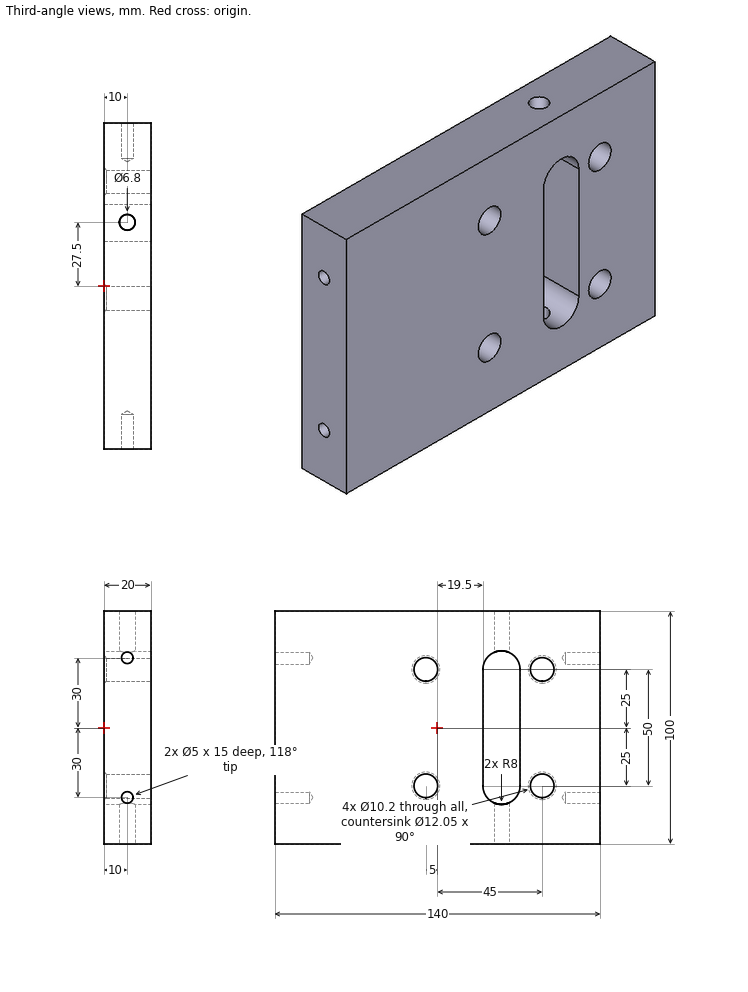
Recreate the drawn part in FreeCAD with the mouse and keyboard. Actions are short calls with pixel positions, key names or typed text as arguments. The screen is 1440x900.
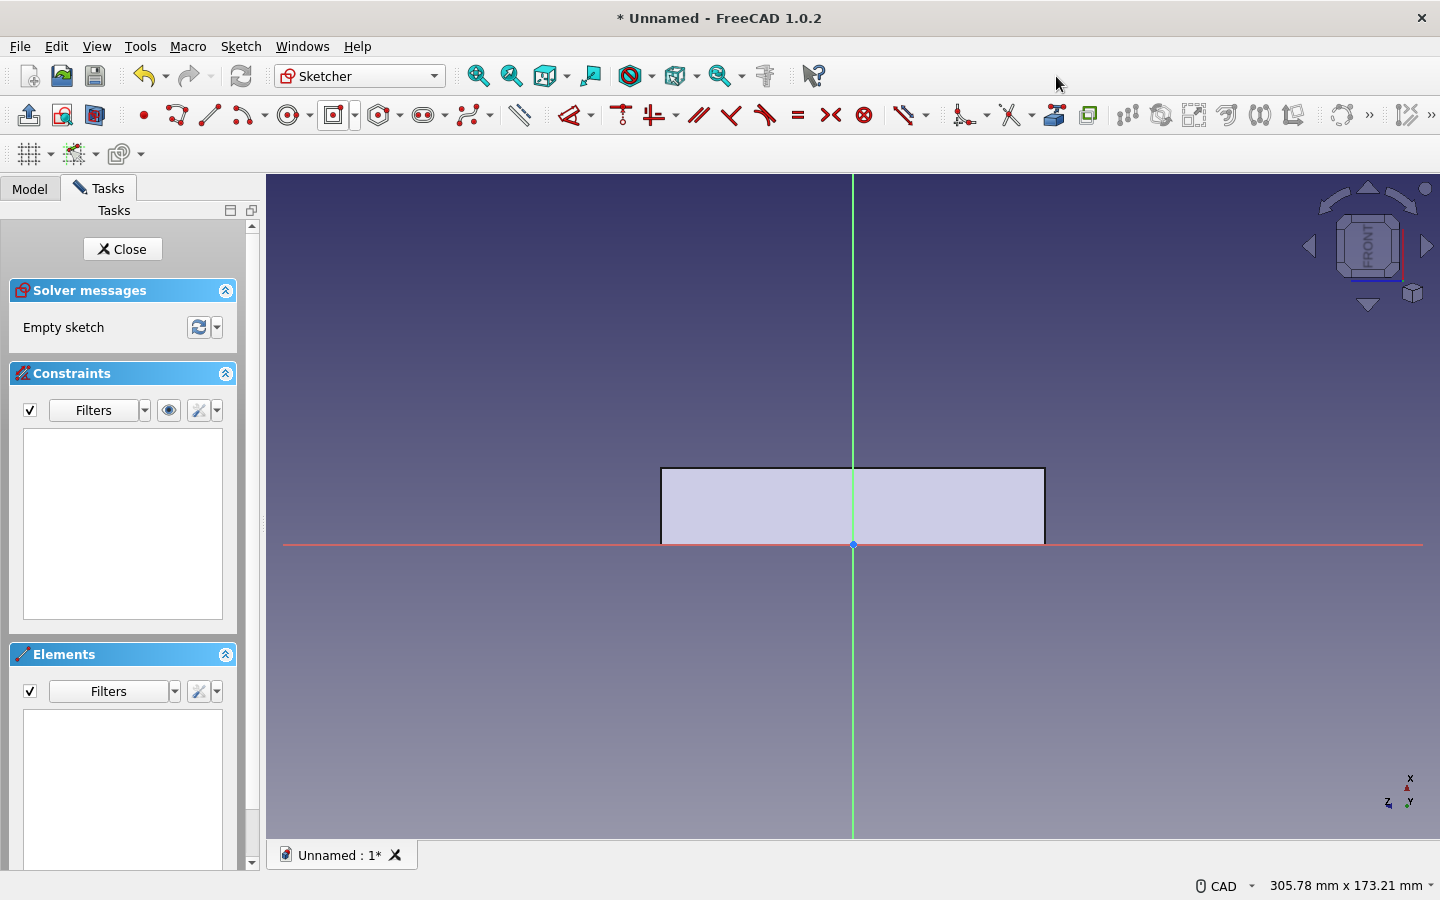
scroll(893, 529, up, 5)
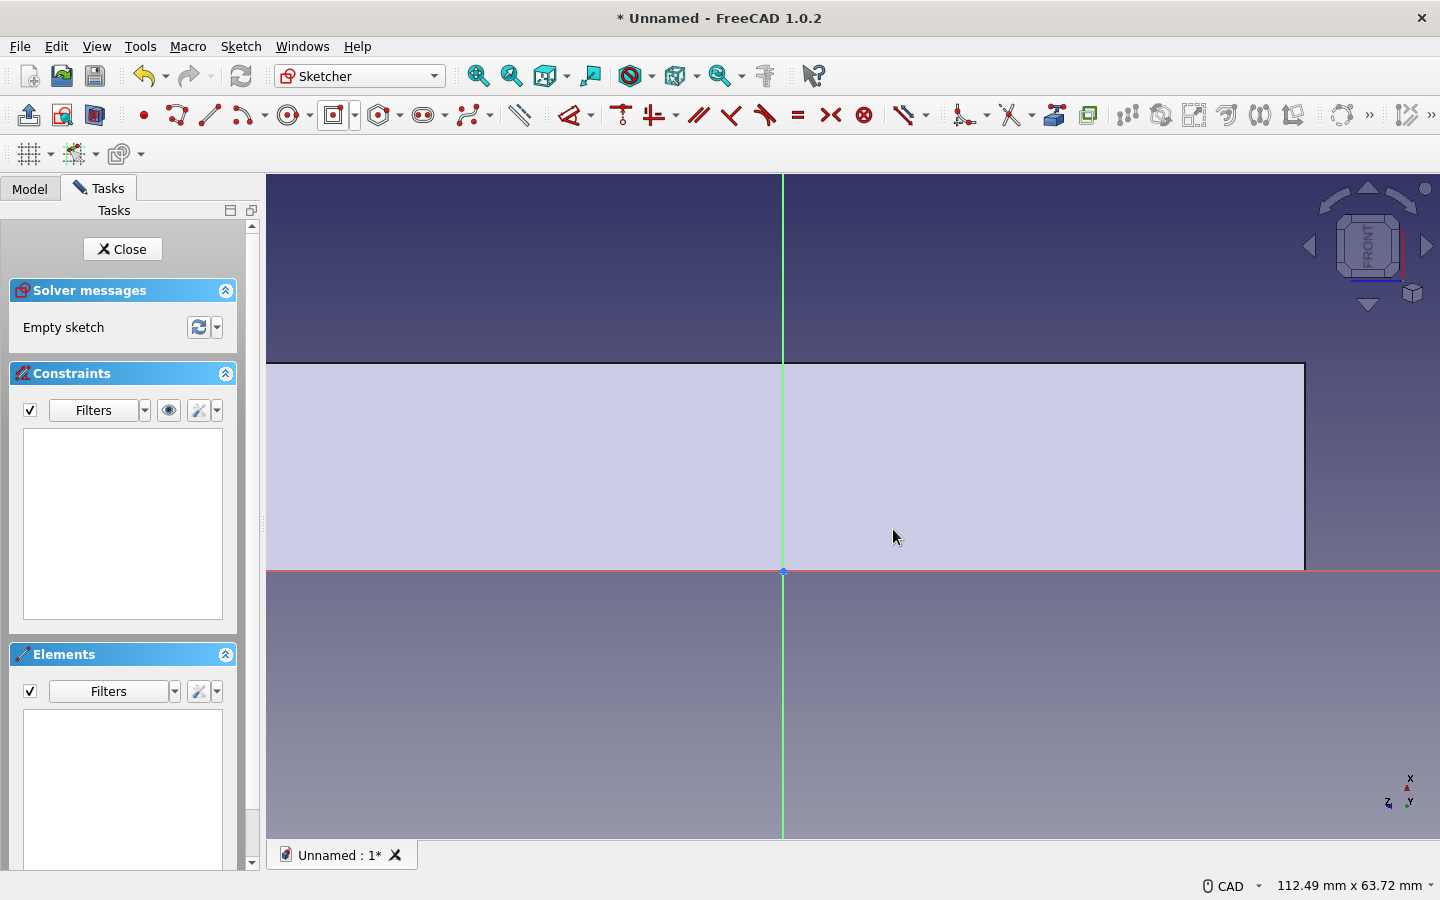
click(288, 116)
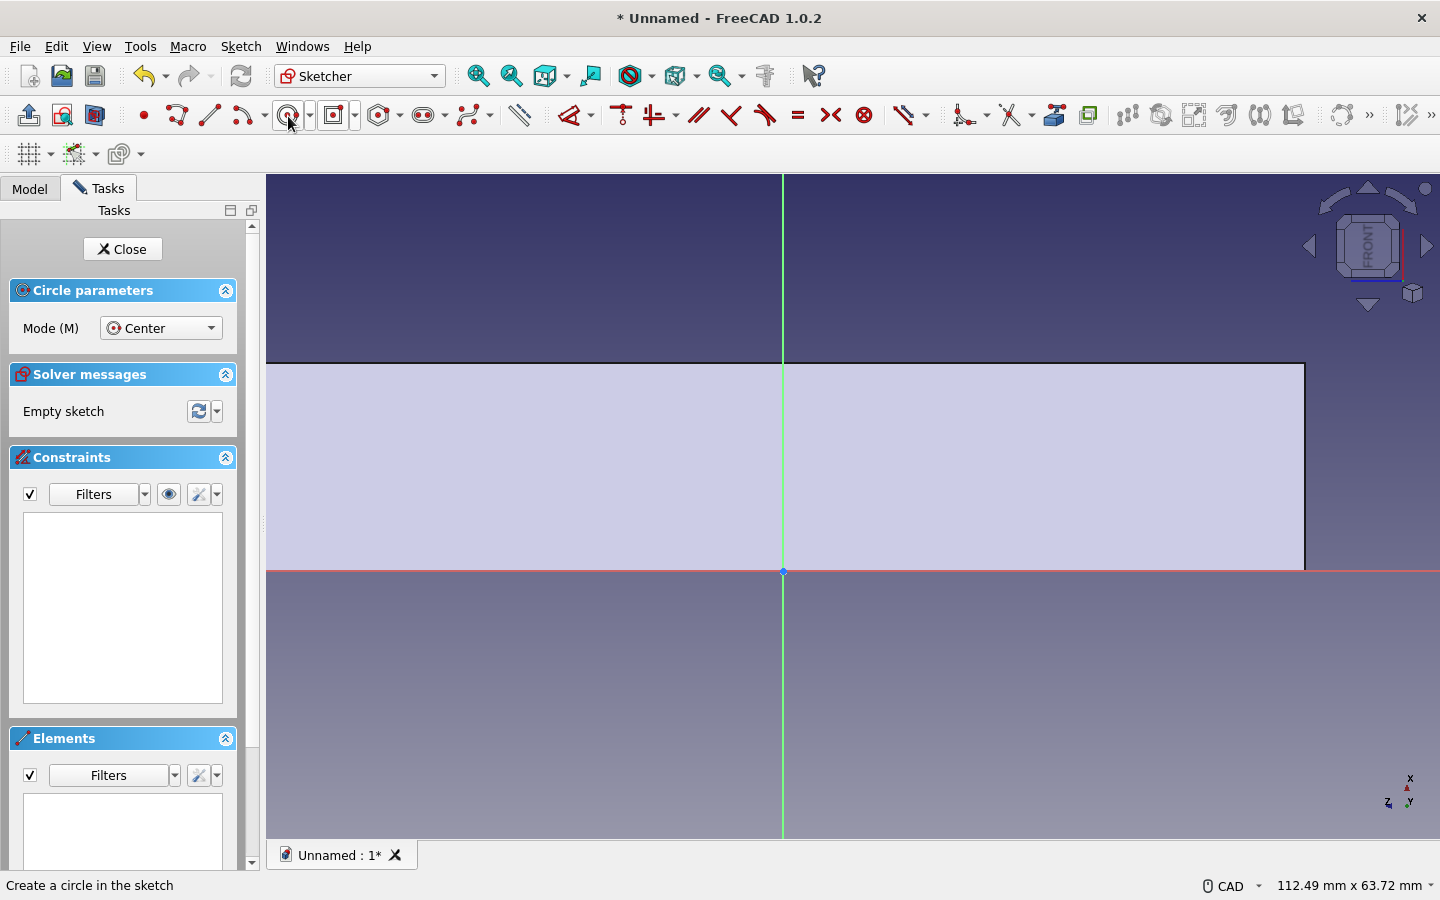
click(1096, 467)
move(1115, 448)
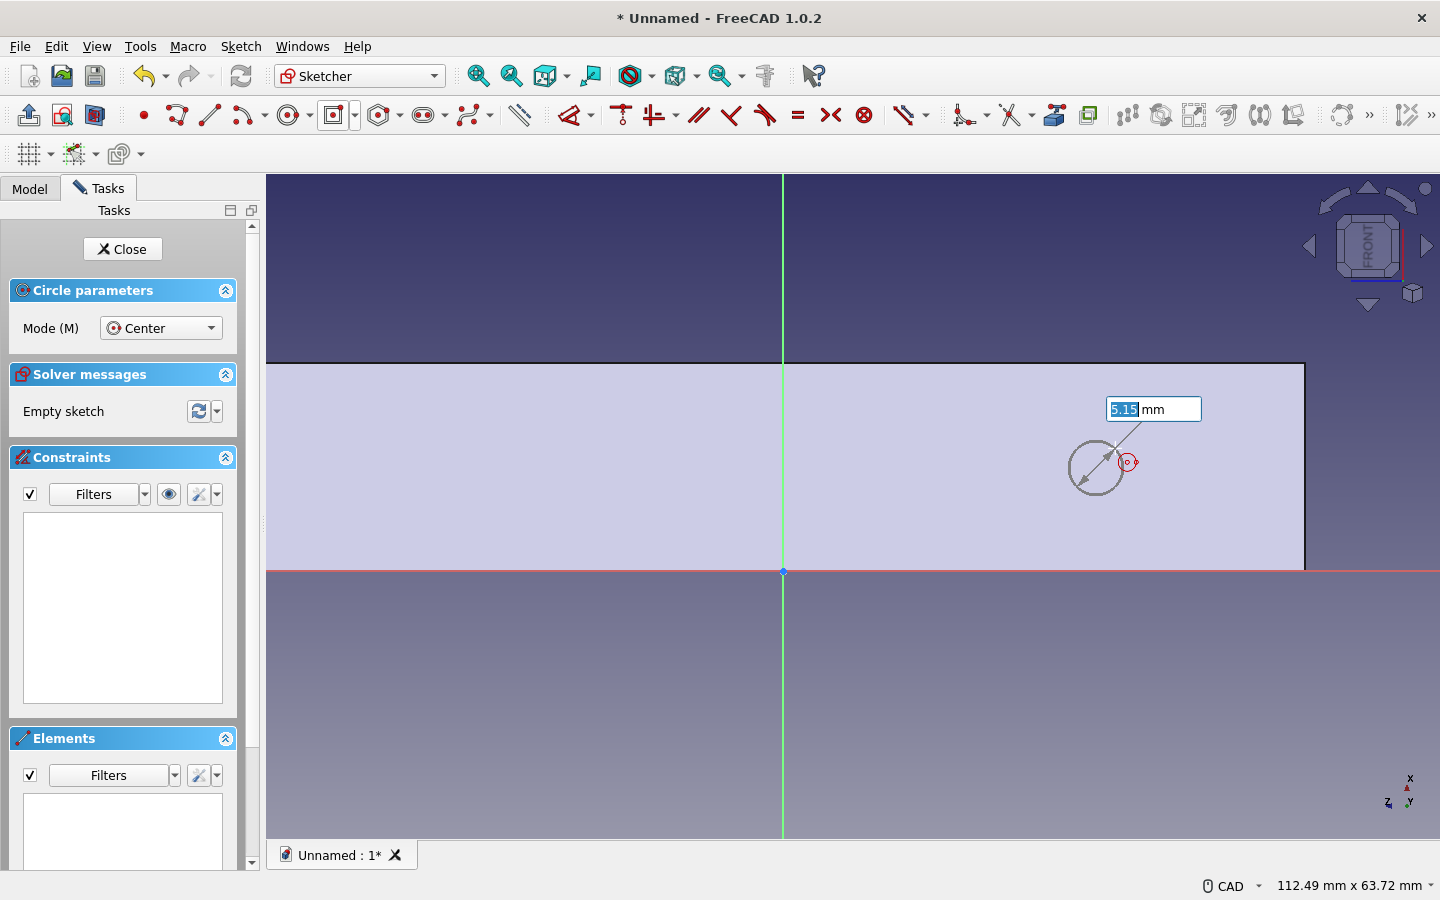
text(5)
key(Return)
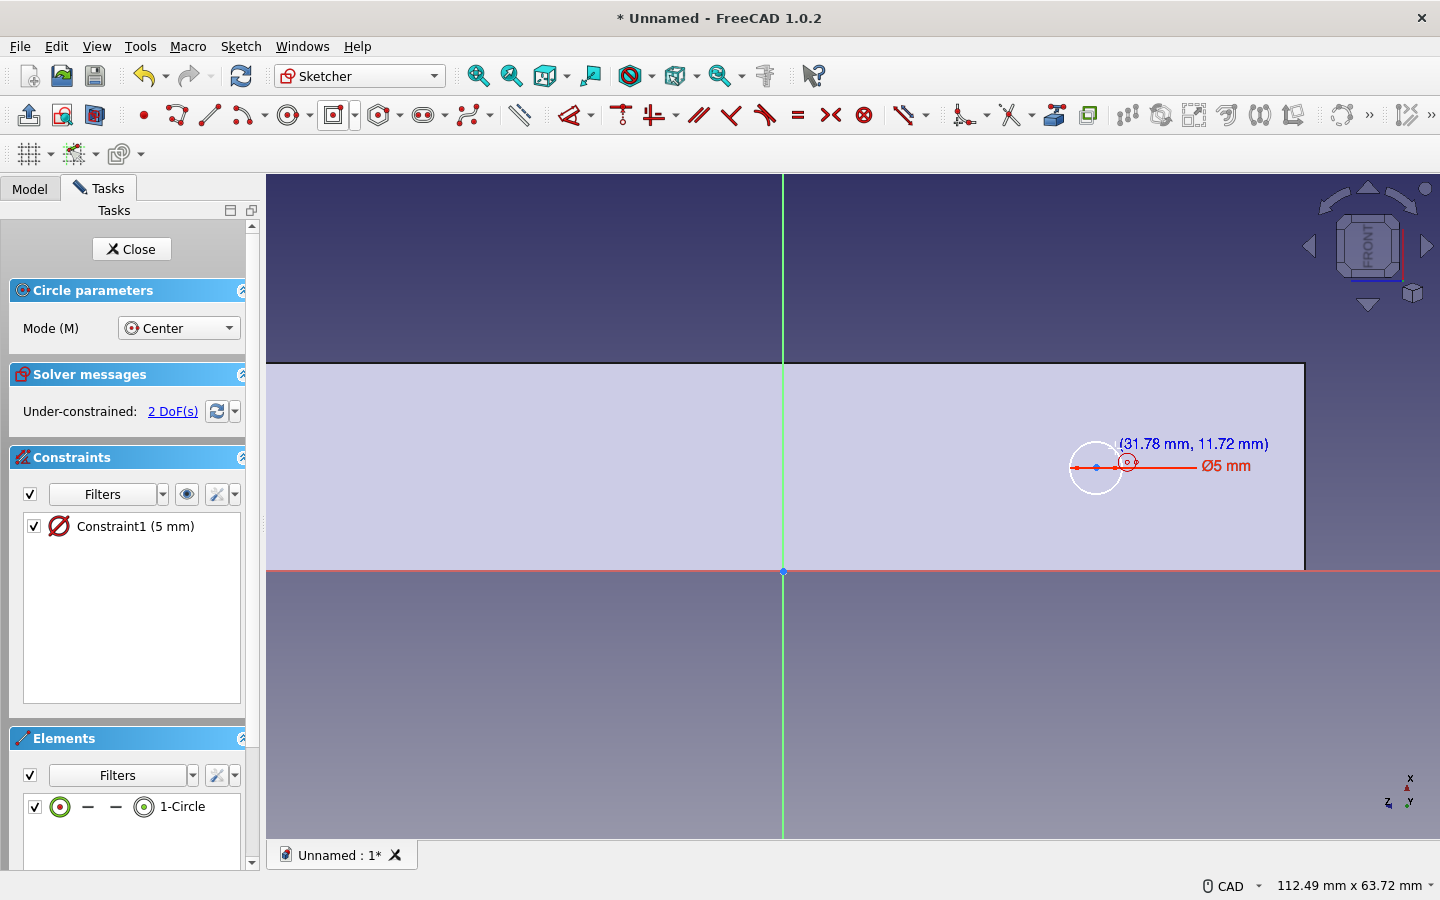
click(470, 467)
move(489, 448)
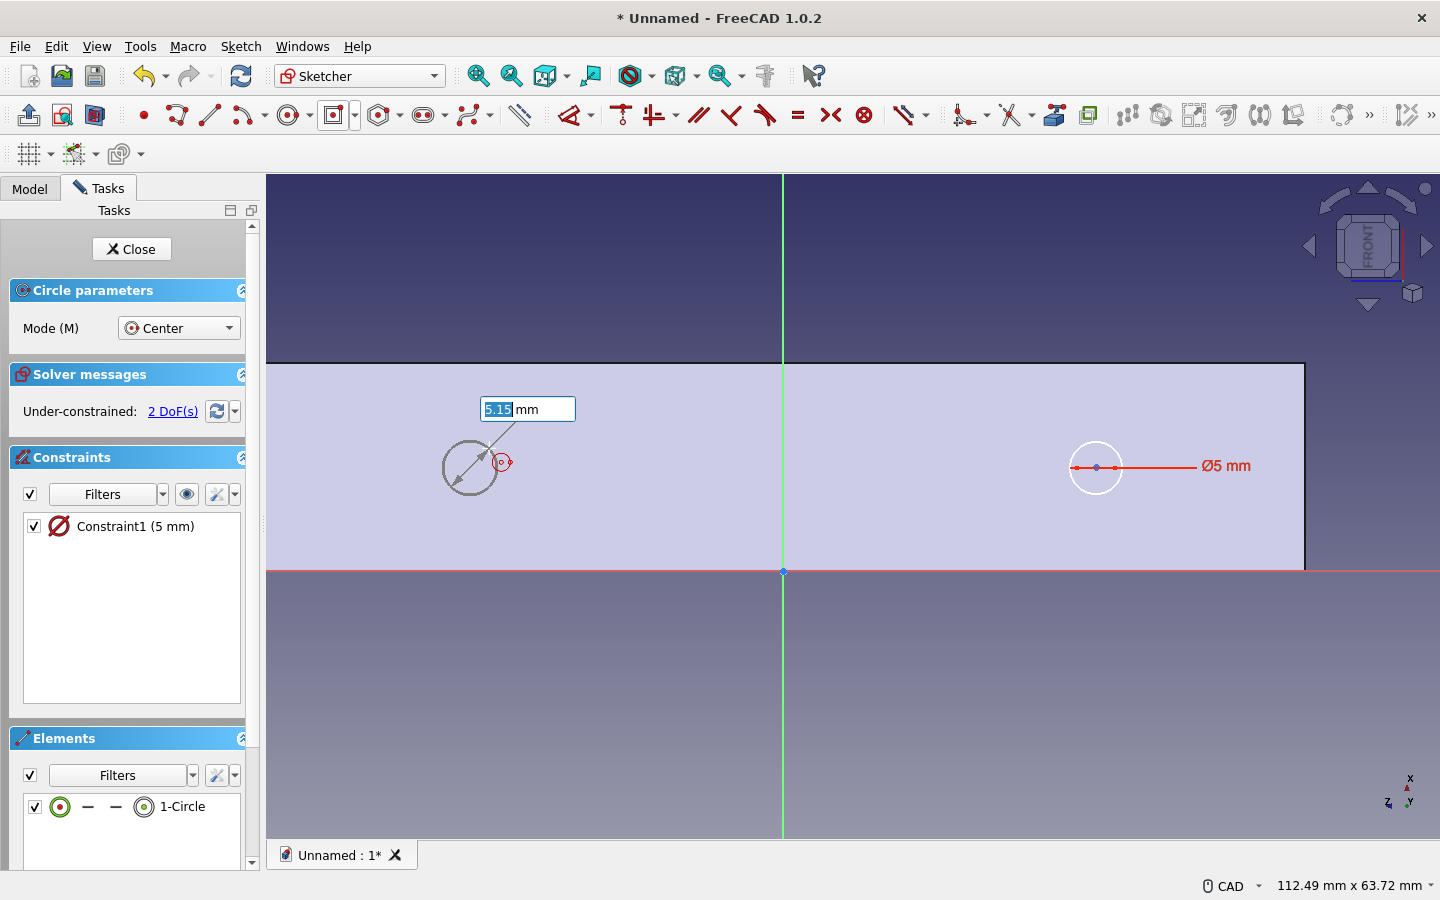
text(5)
key(Return)
key(Escape)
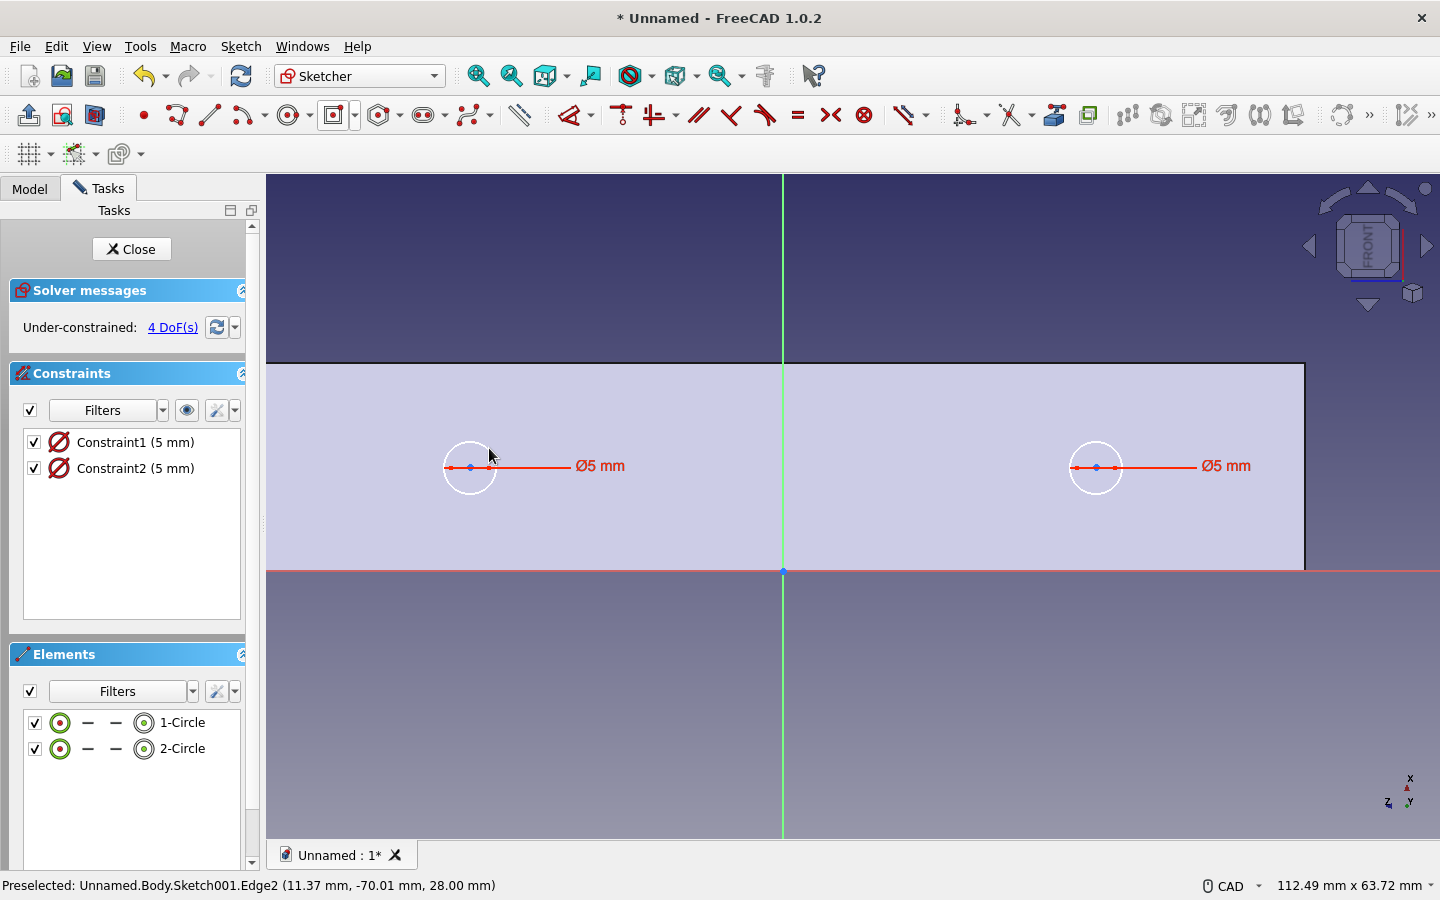
click(1096, 468)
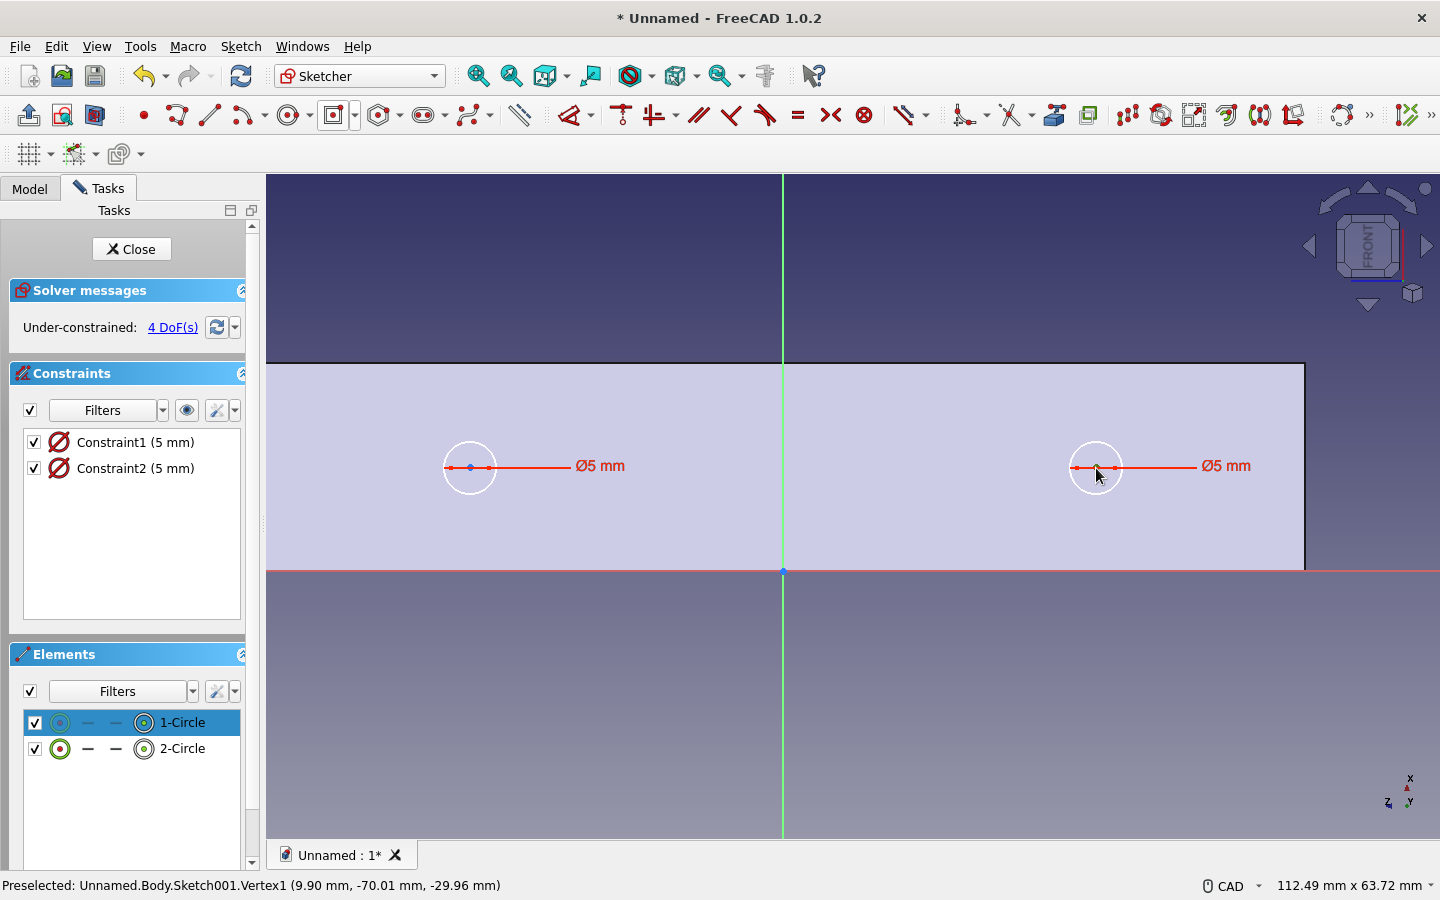
click(470, 468)